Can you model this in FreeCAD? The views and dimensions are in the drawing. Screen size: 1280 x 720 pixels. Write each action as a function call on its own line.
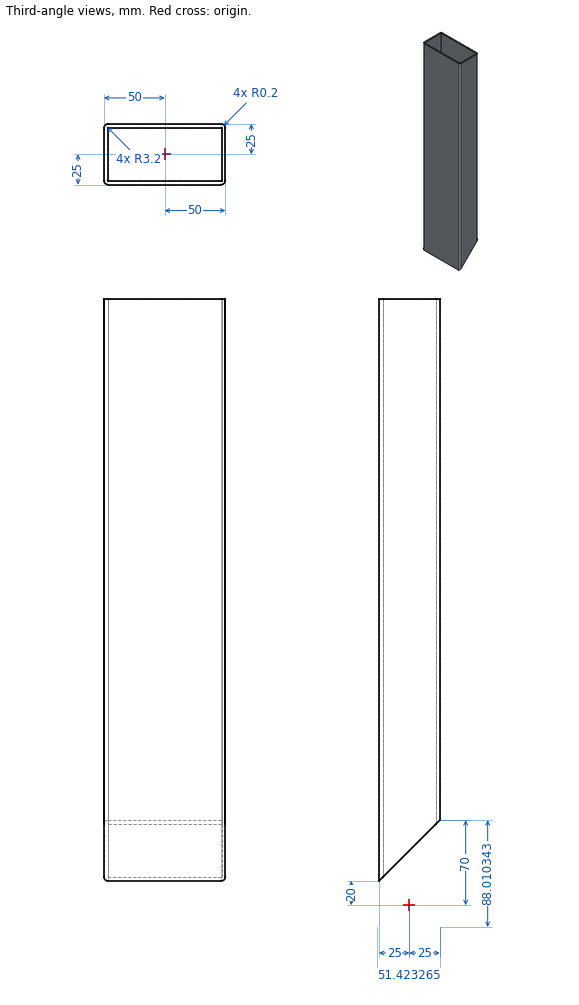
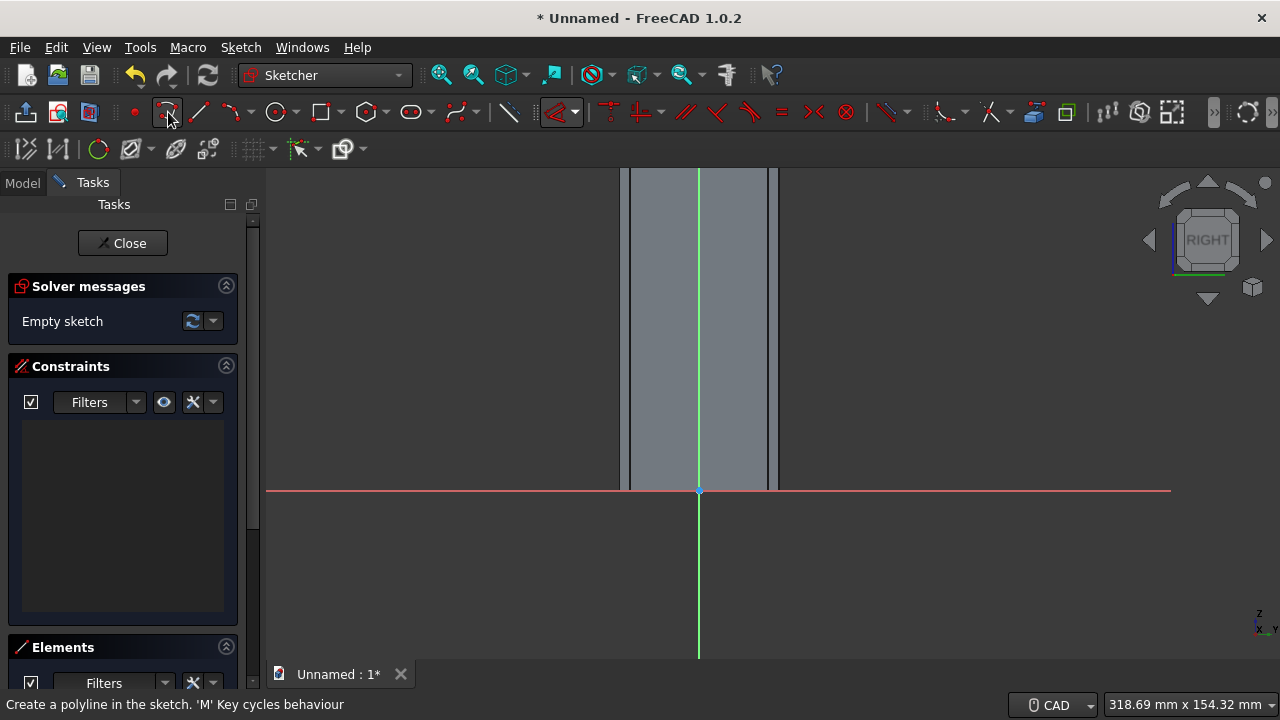
click(779, 548)
click(779, 268)
click(620, 427)
click(613, 548)
click(779, 549)
key(Escape)
key(Escape)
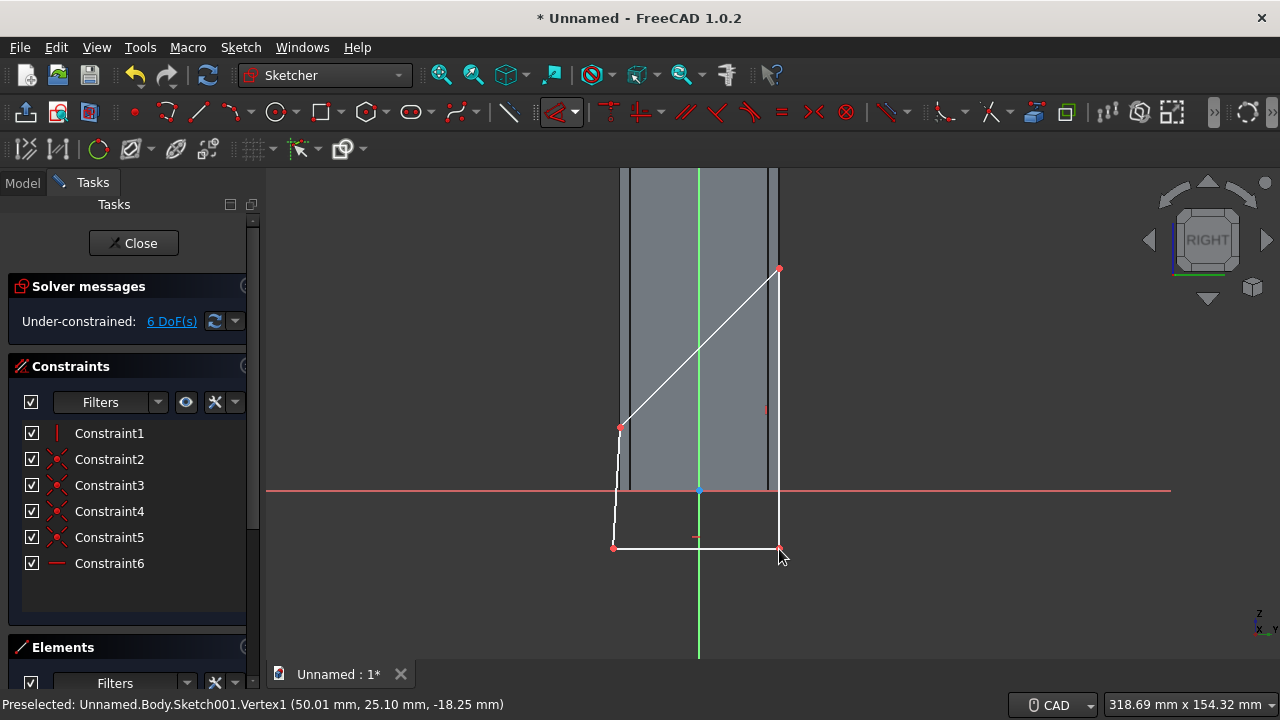
click(779, 549)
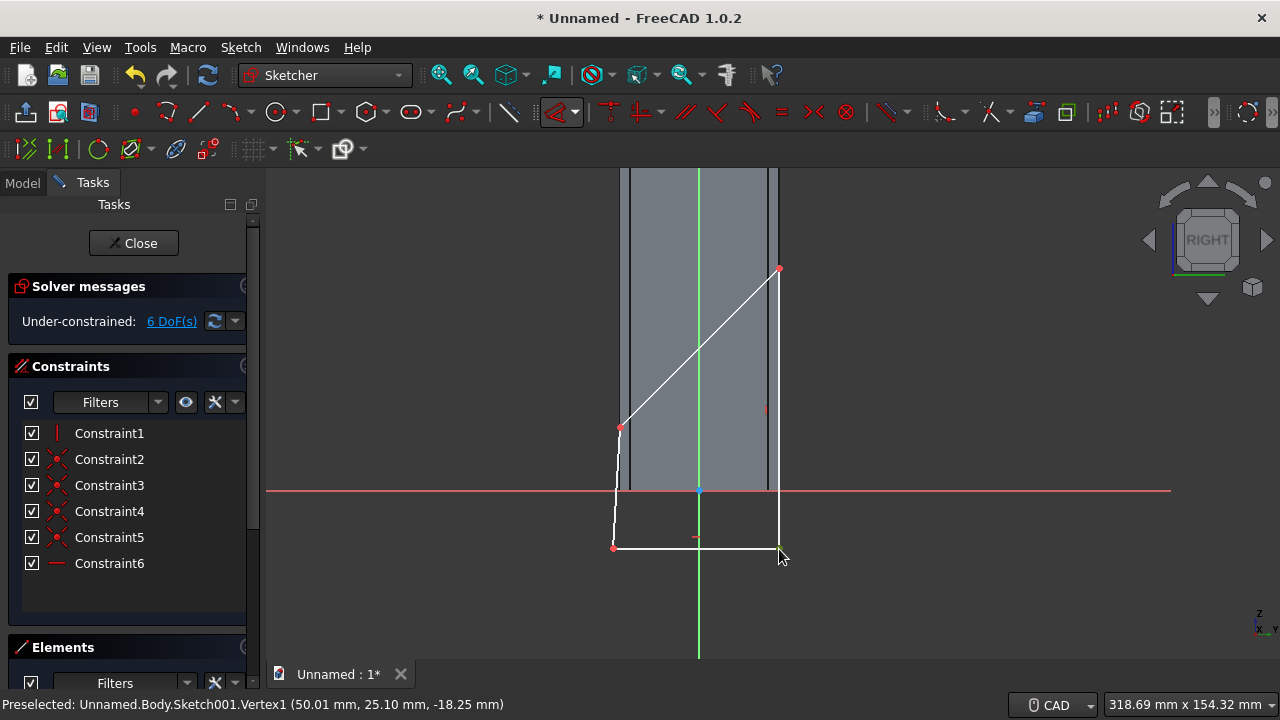
click(578, 112)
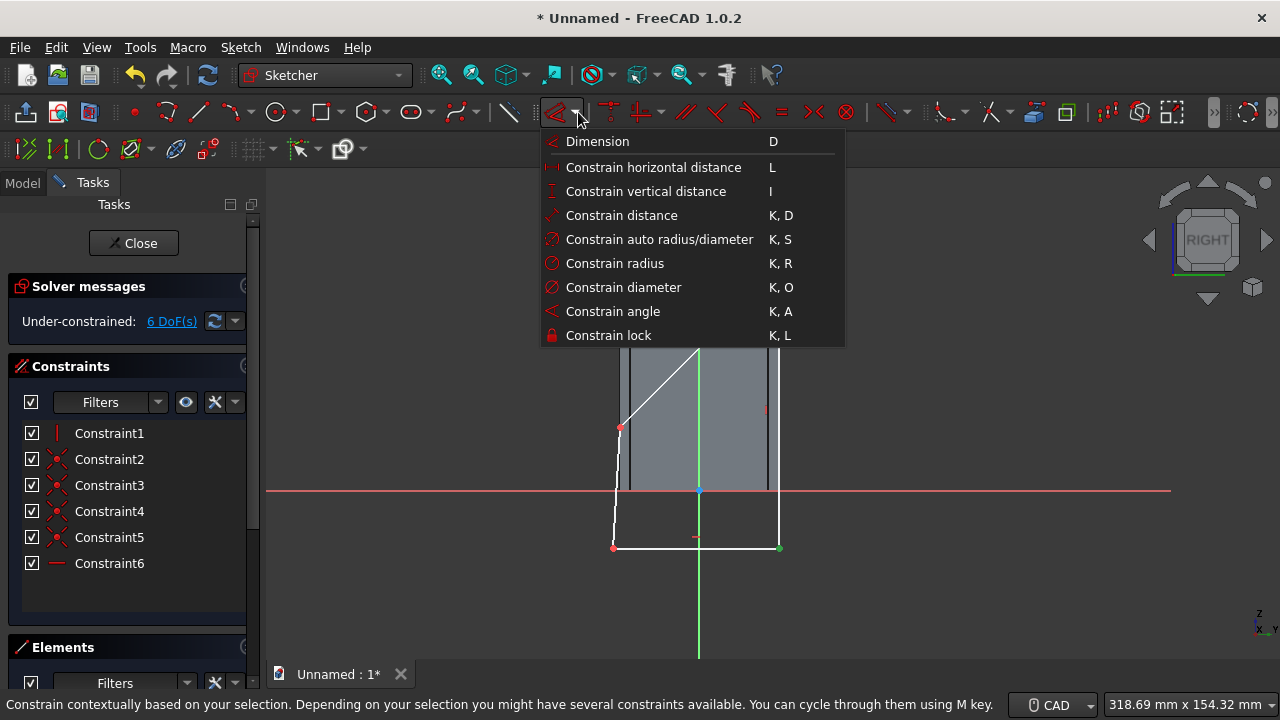
click(693, 167)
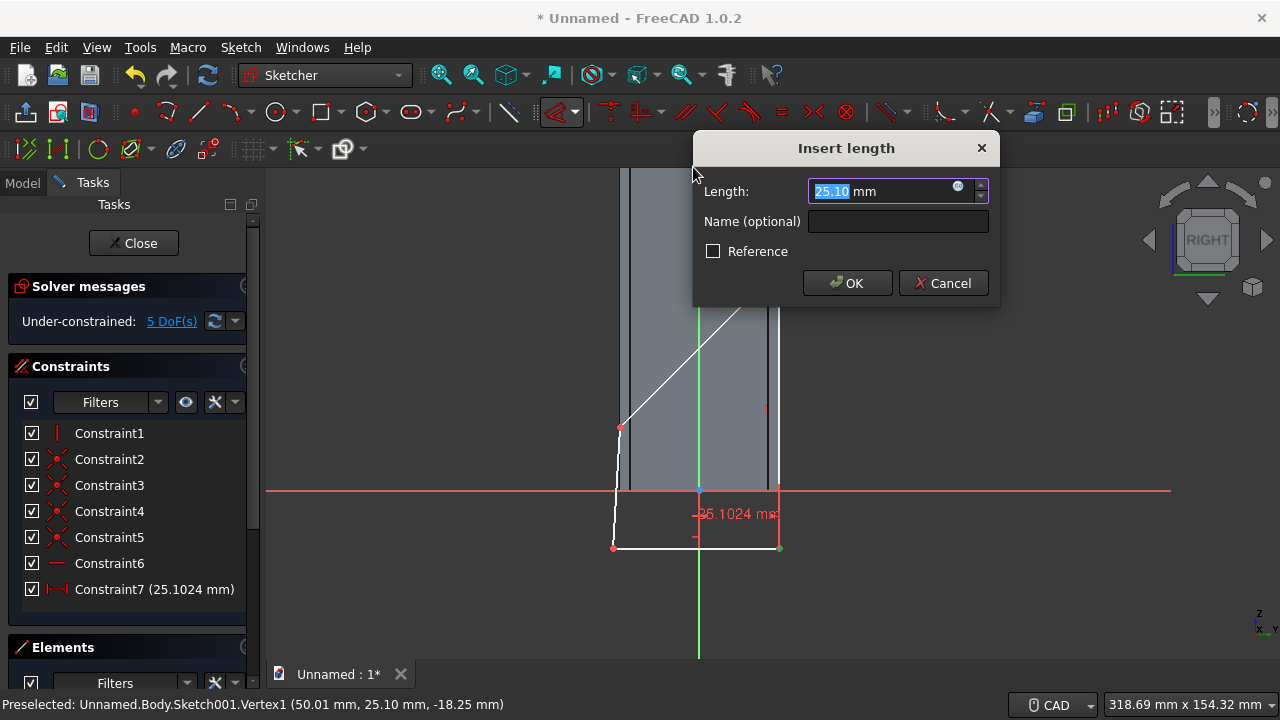
text(25)
key(Return)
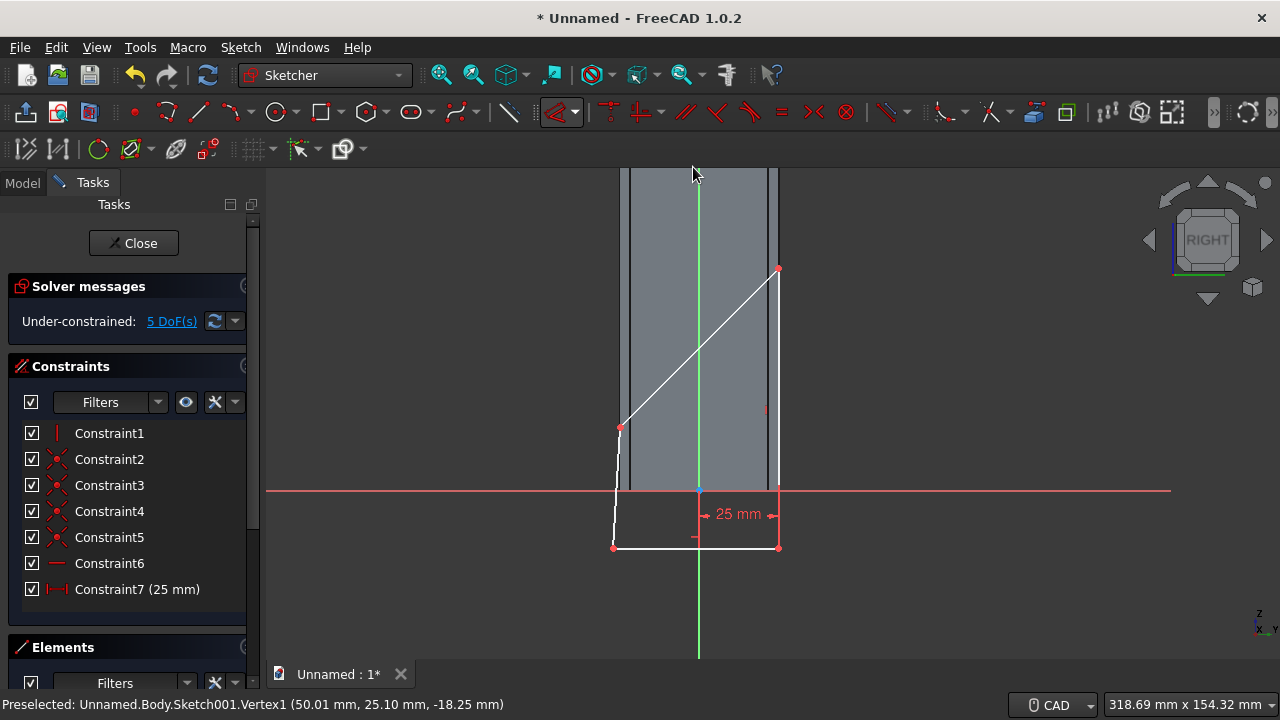
click(779, 269)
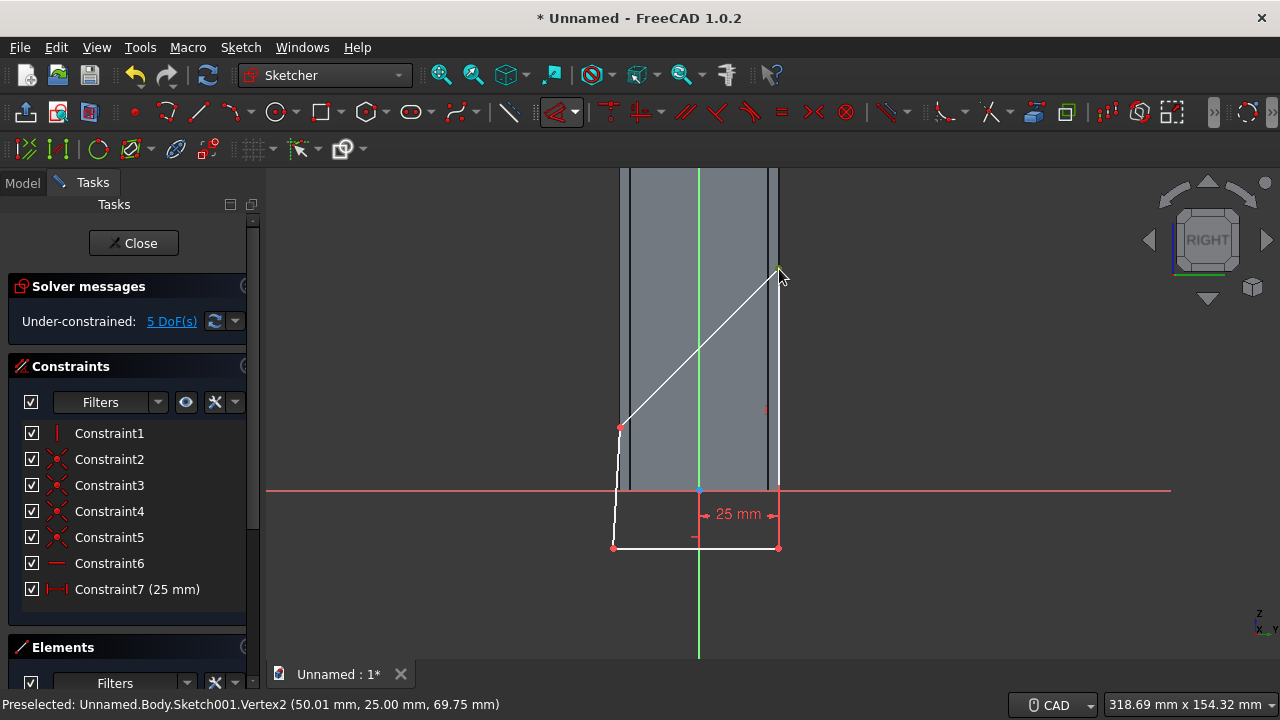
key(i)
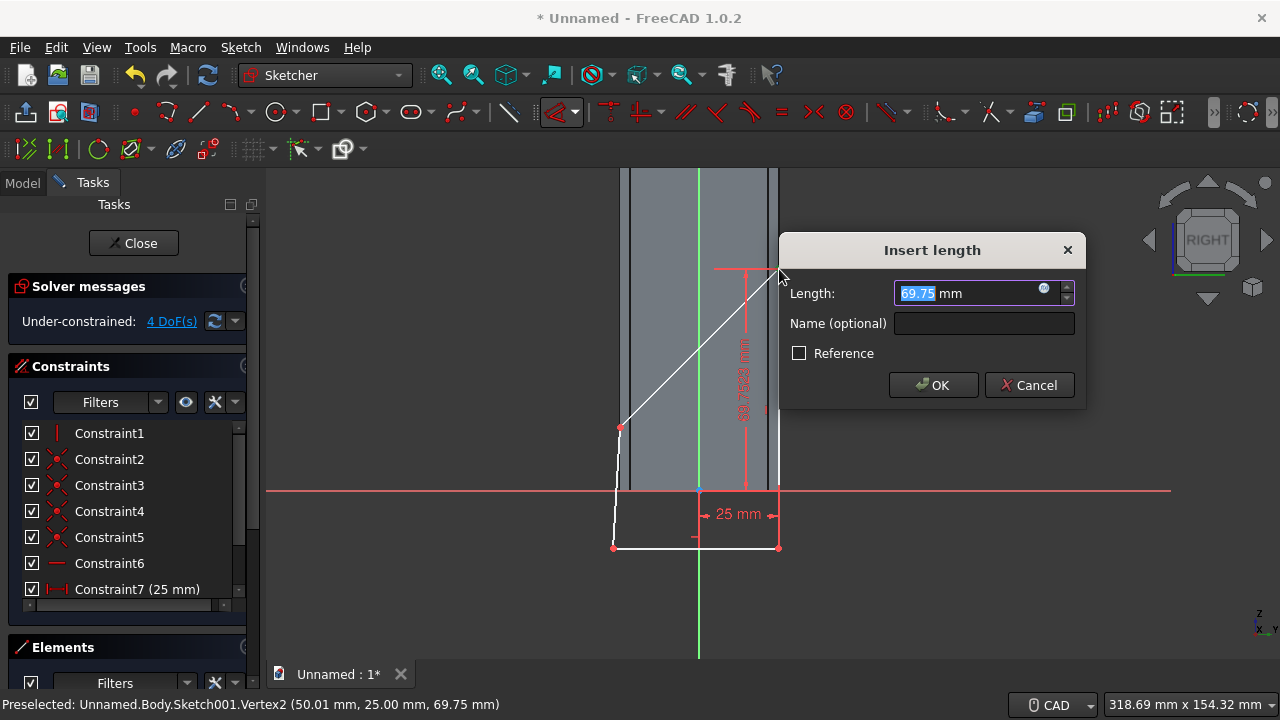
text(70)
key(Return)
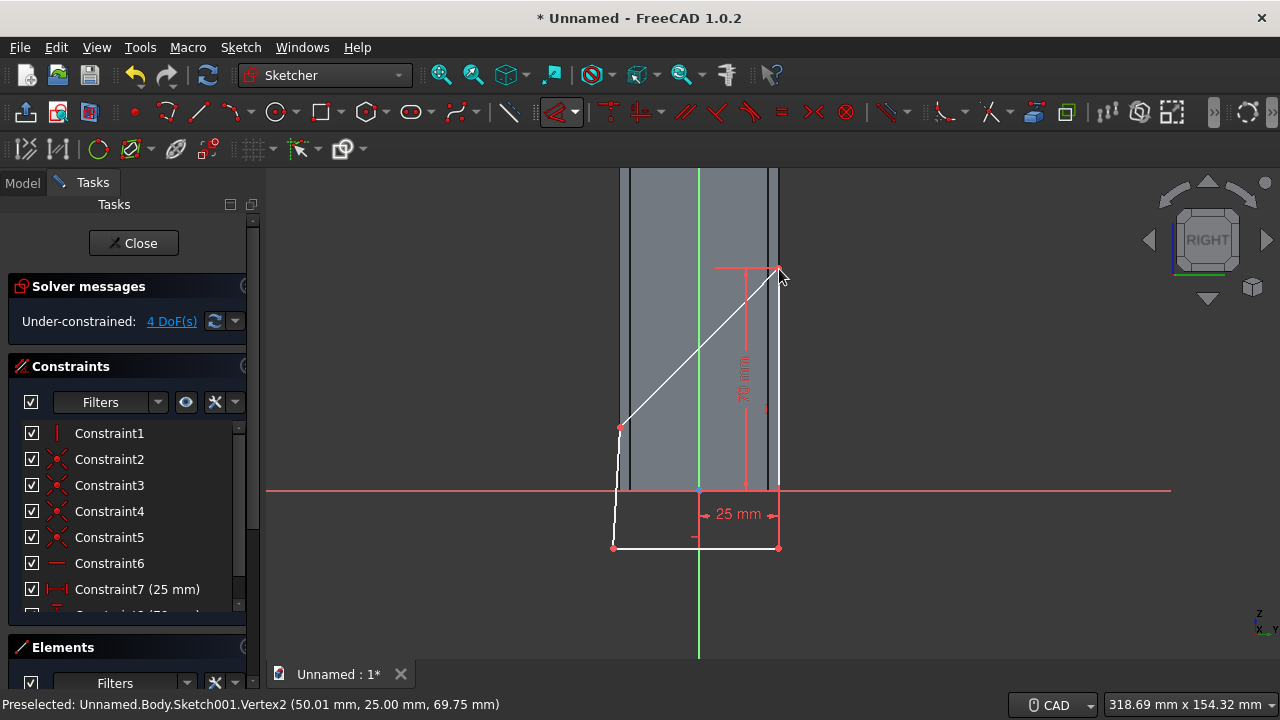
click(620, 428)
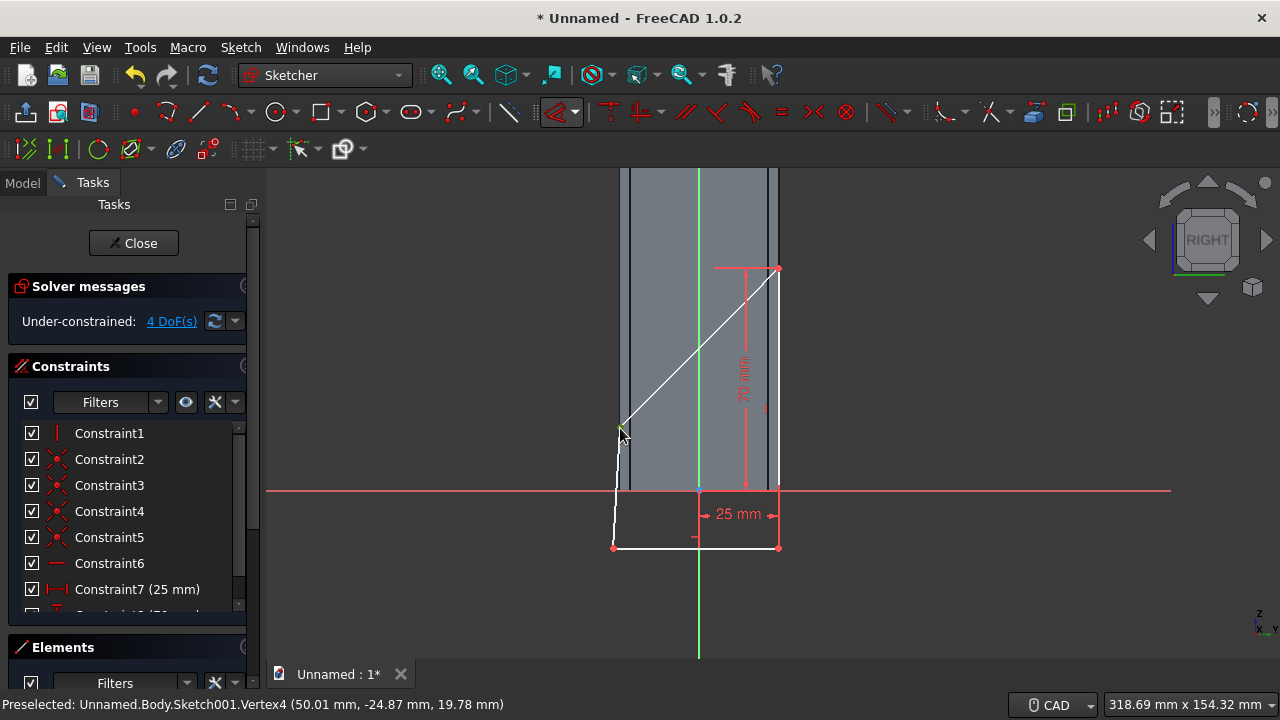
key(l)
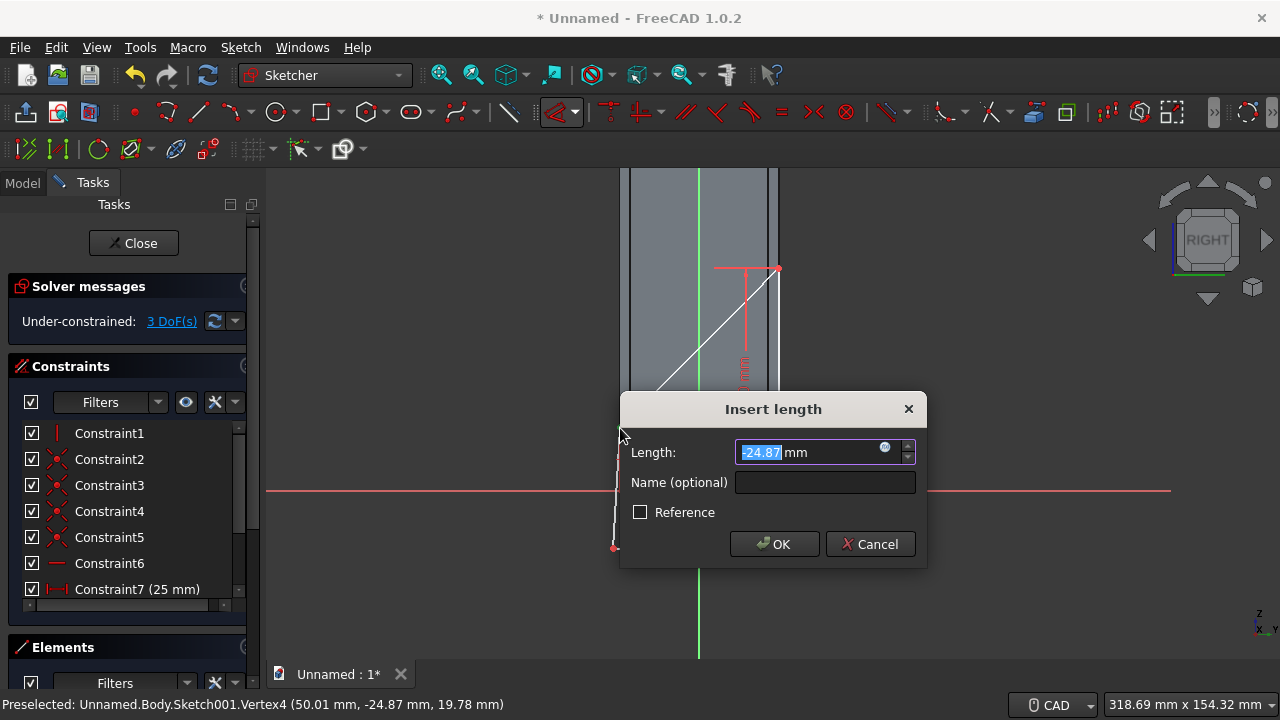
text(-25)
key(Return)